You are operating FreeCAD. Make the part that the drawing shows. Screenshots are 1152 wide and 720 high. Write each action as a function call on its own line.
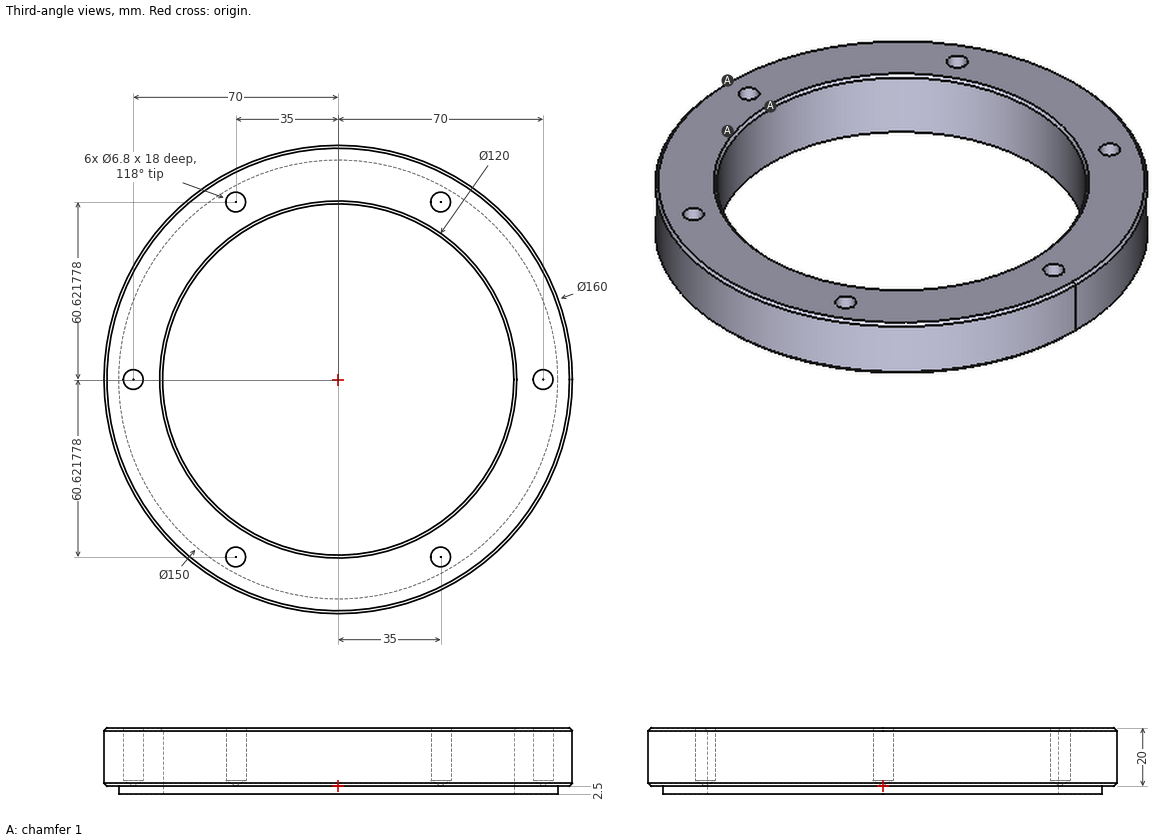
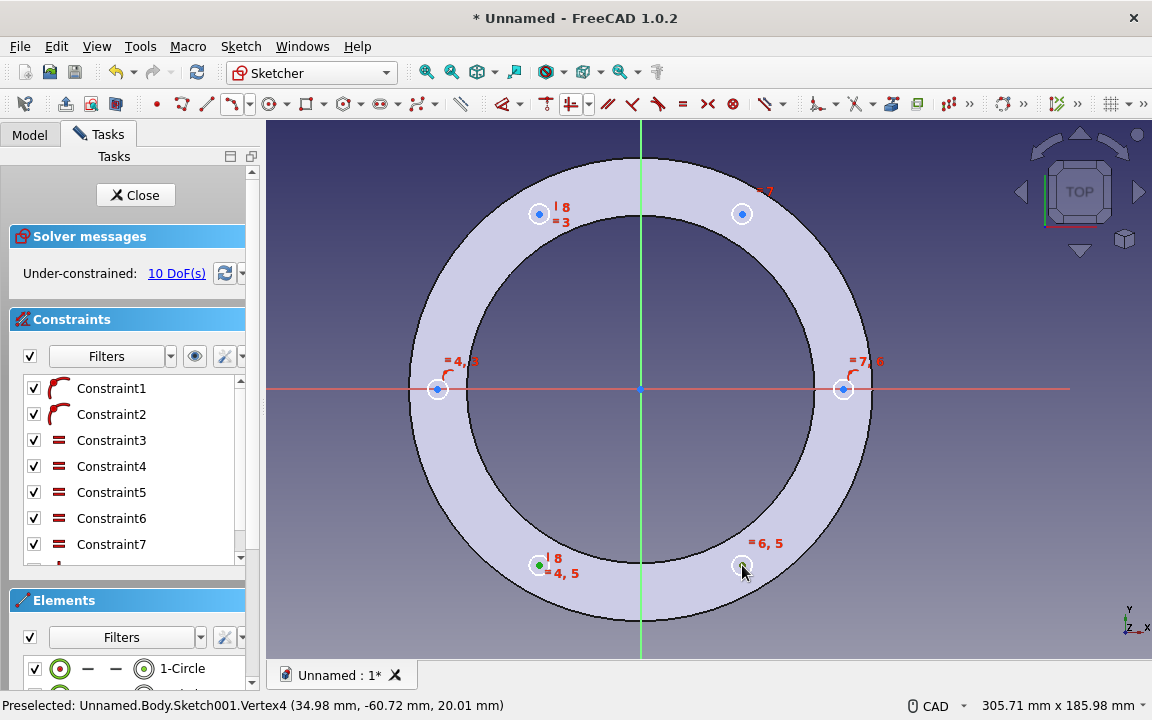
key(h)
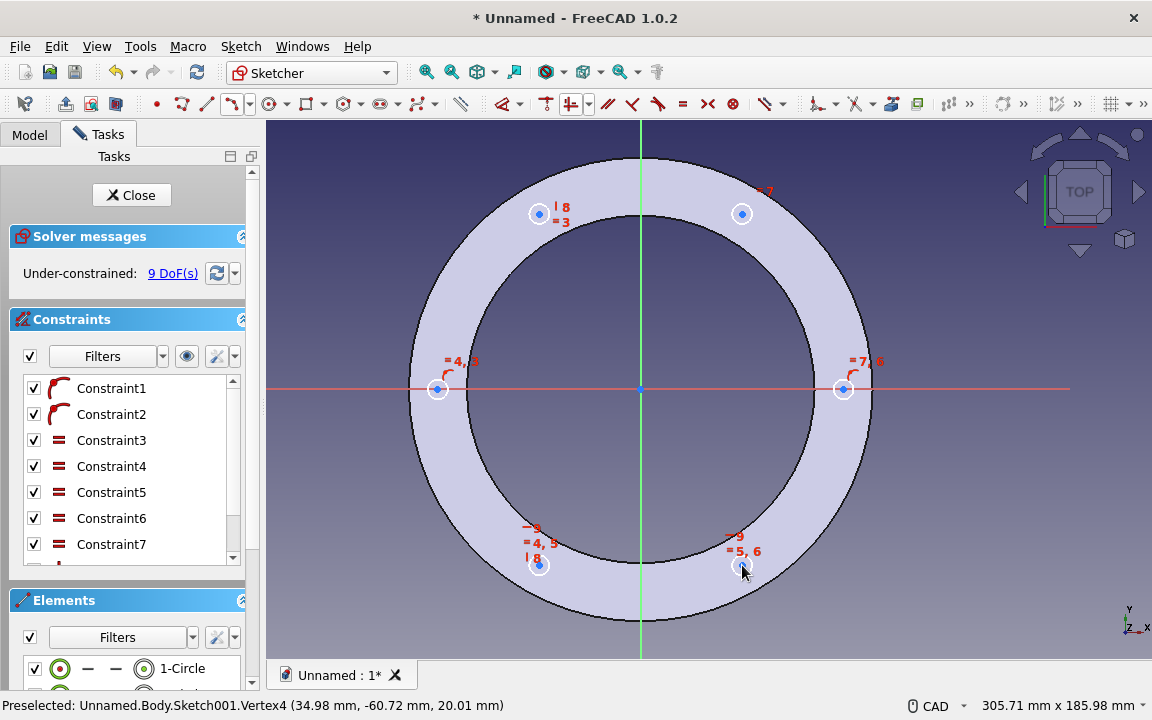
click(742, 565)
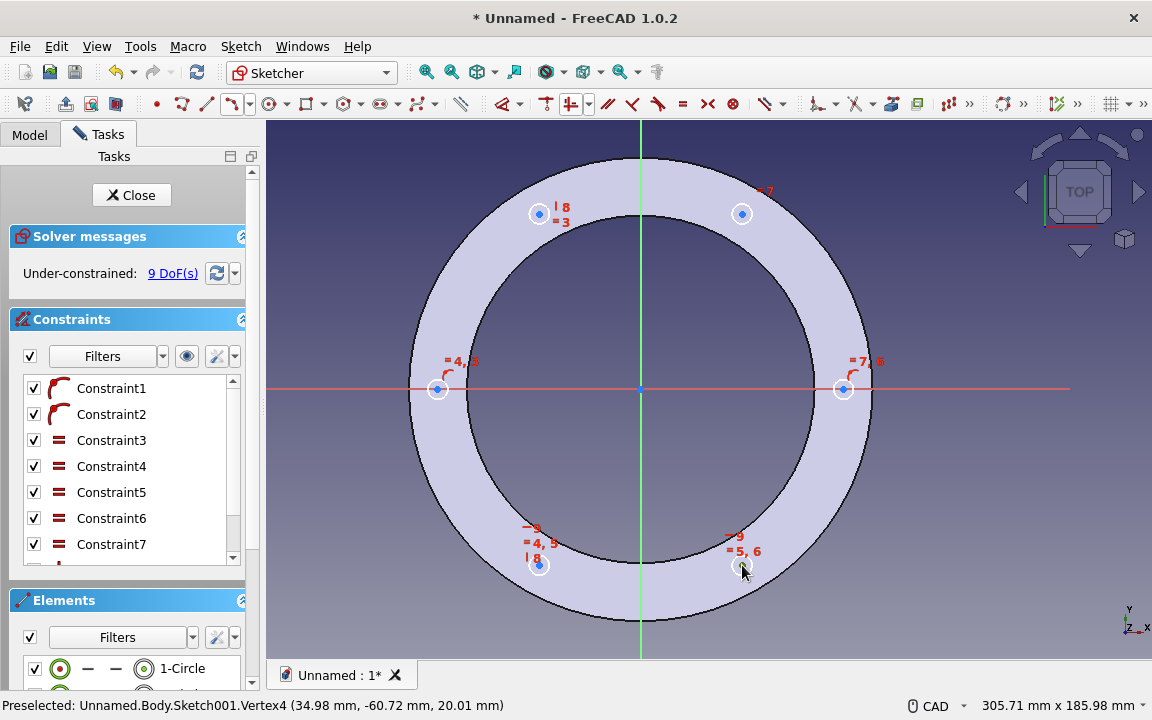
click(742, 214)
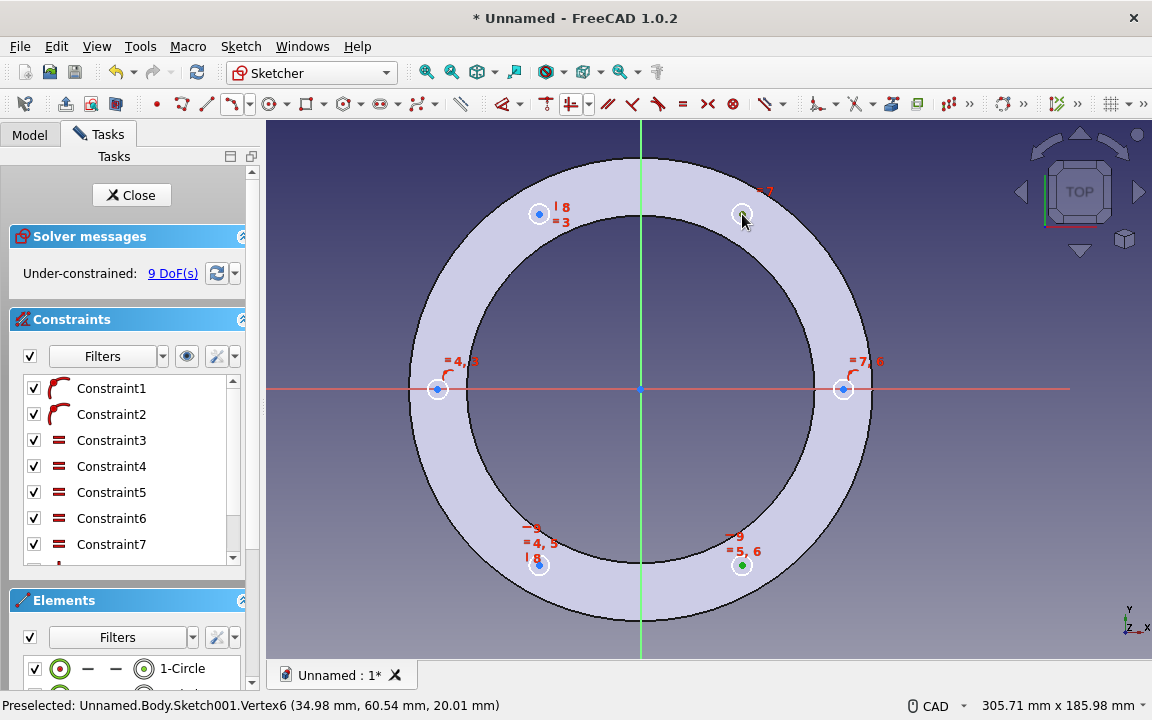
key(v)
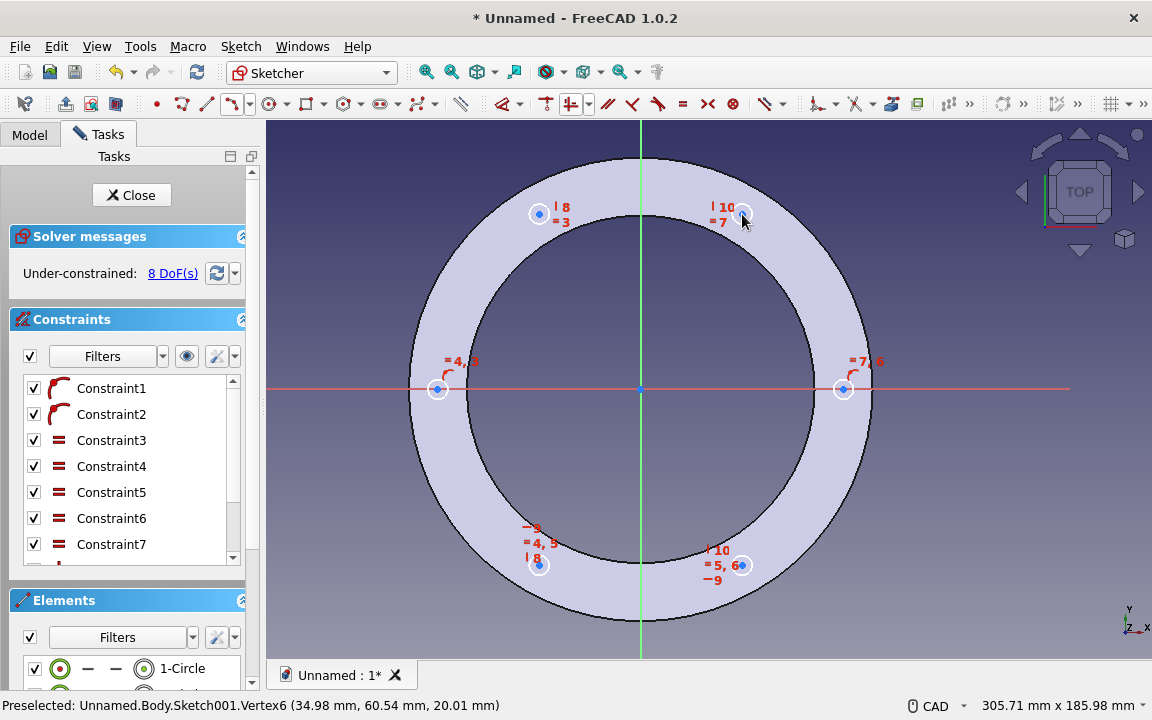
click(539, 214)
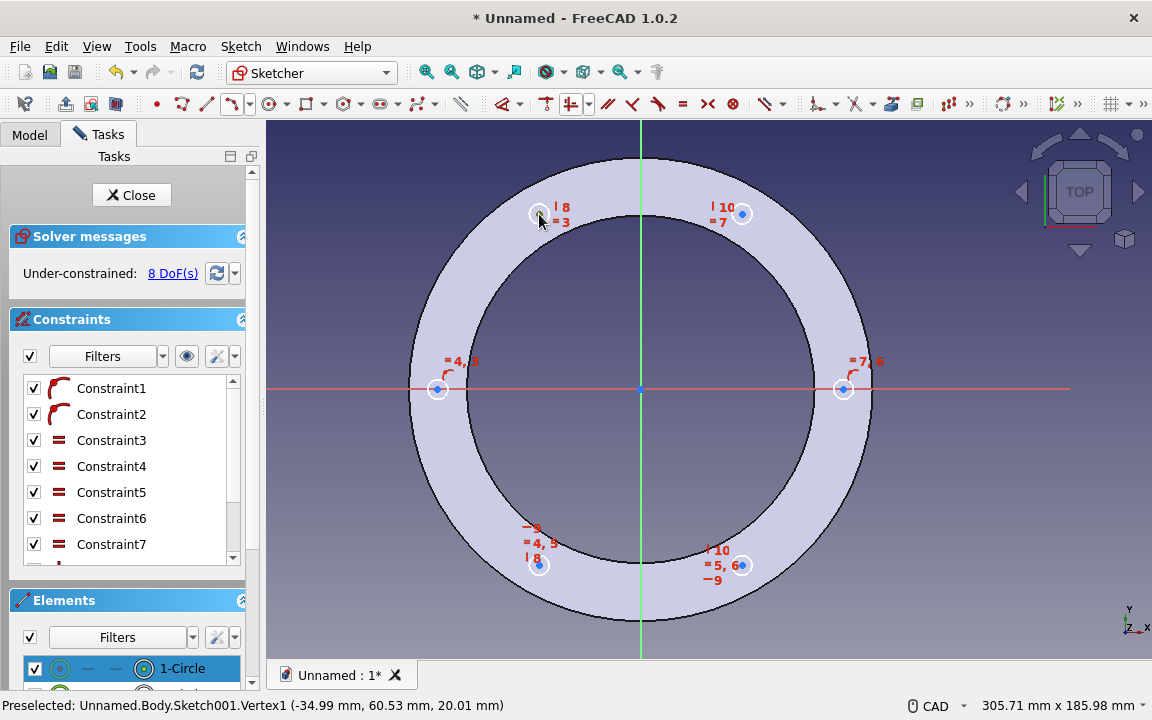
click(742, 214)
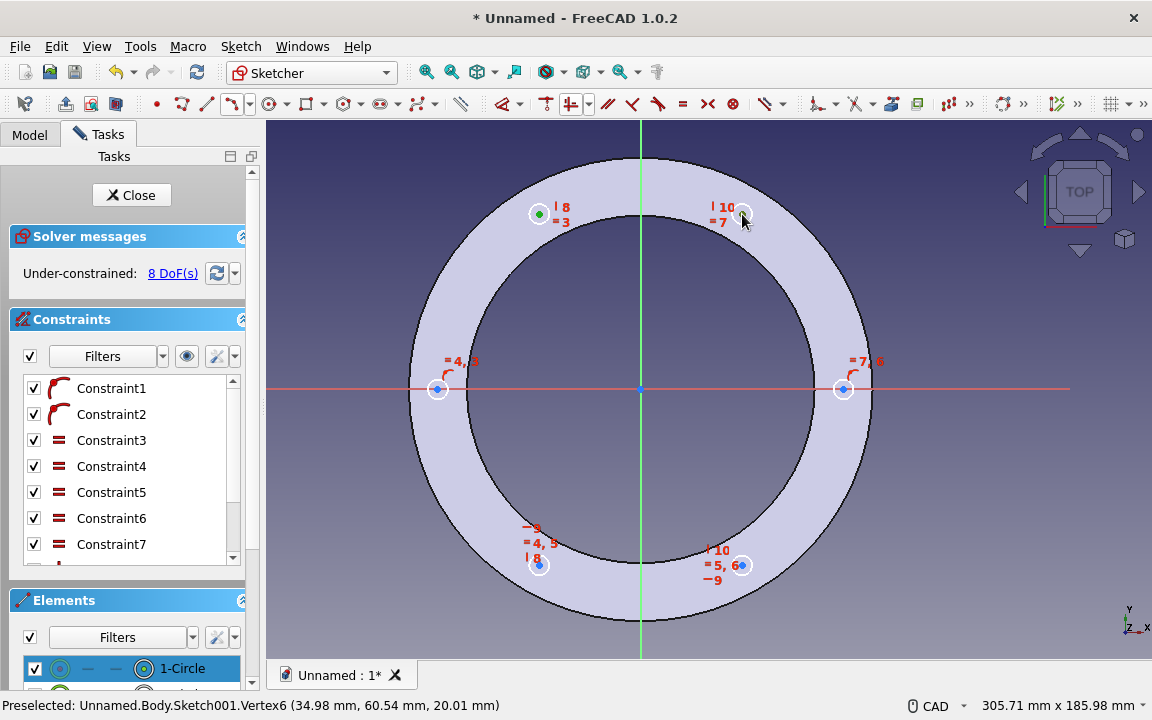
key(h)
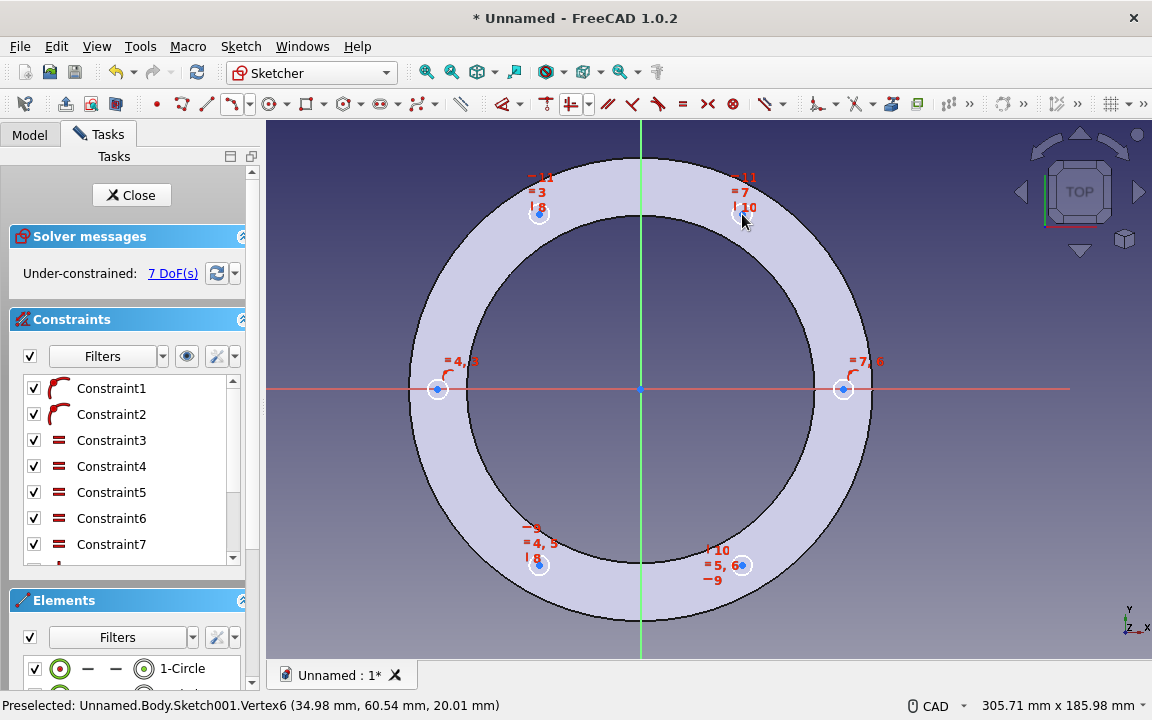
click(502, 104)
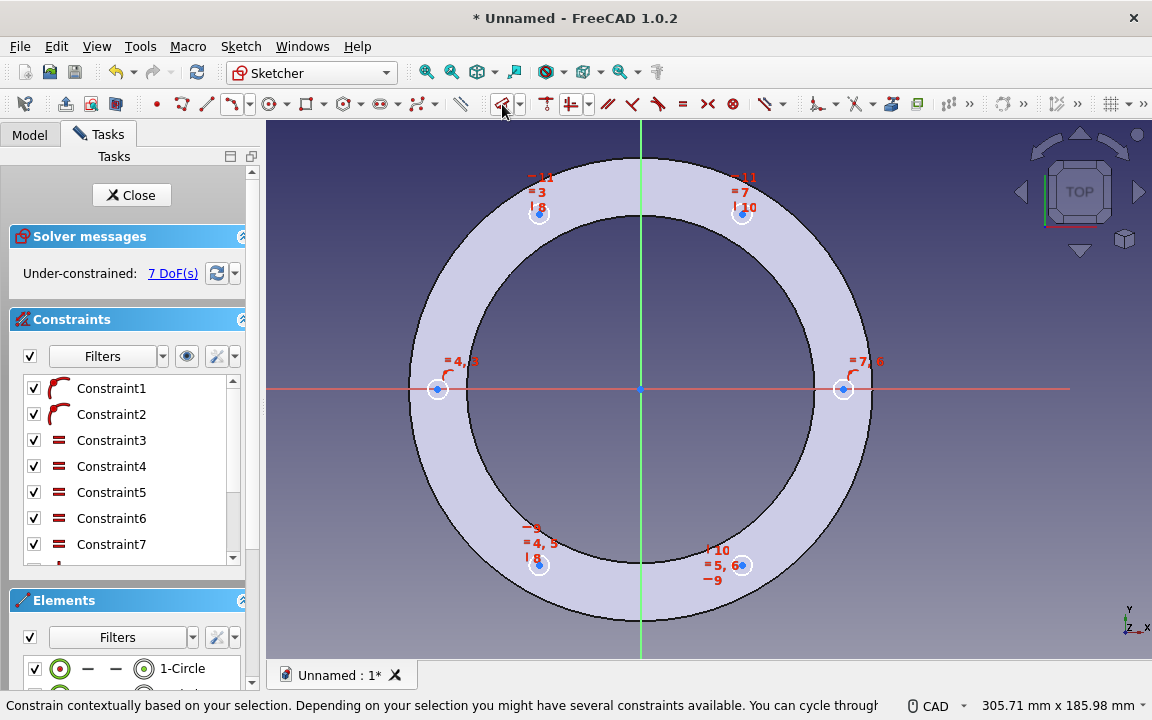
scroll(546, 207, up, 4)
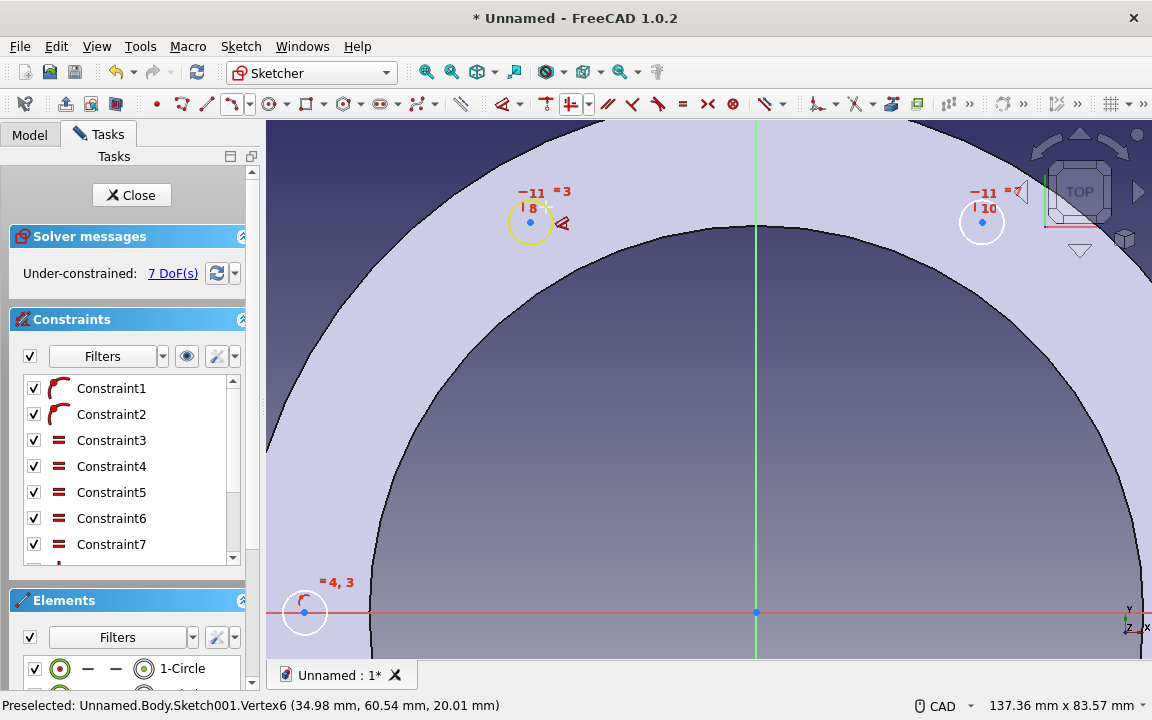
click(546, 207)
click(569, 184)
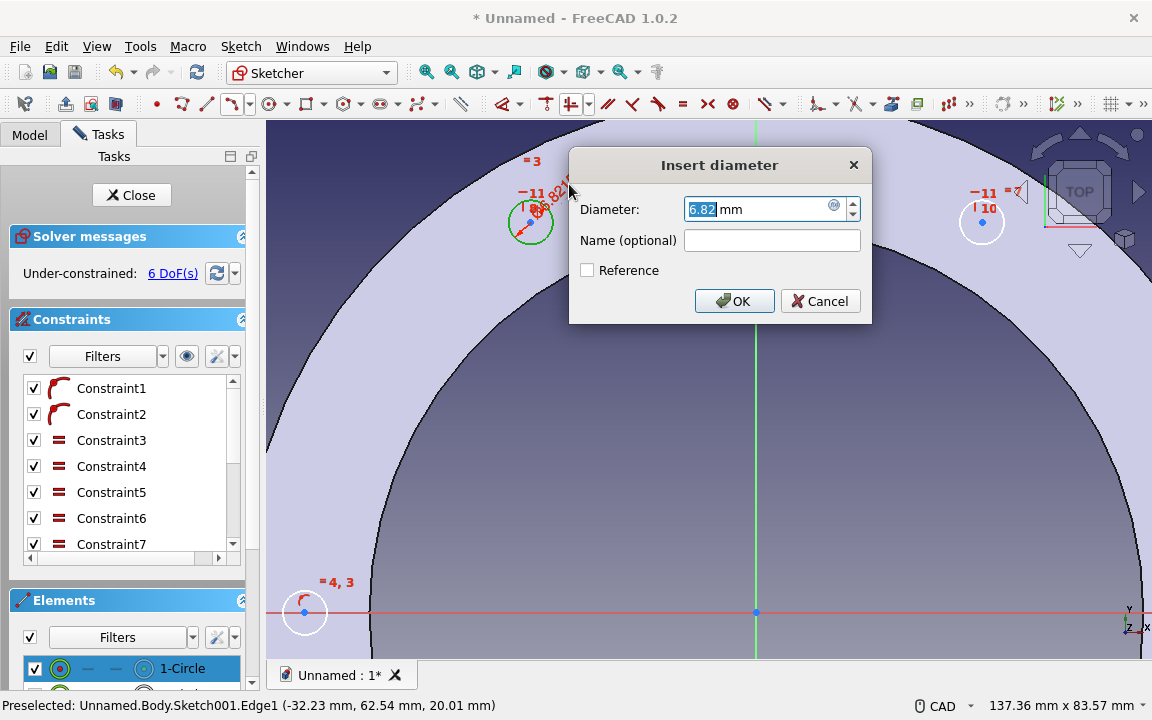
text(6.8)
key(Return)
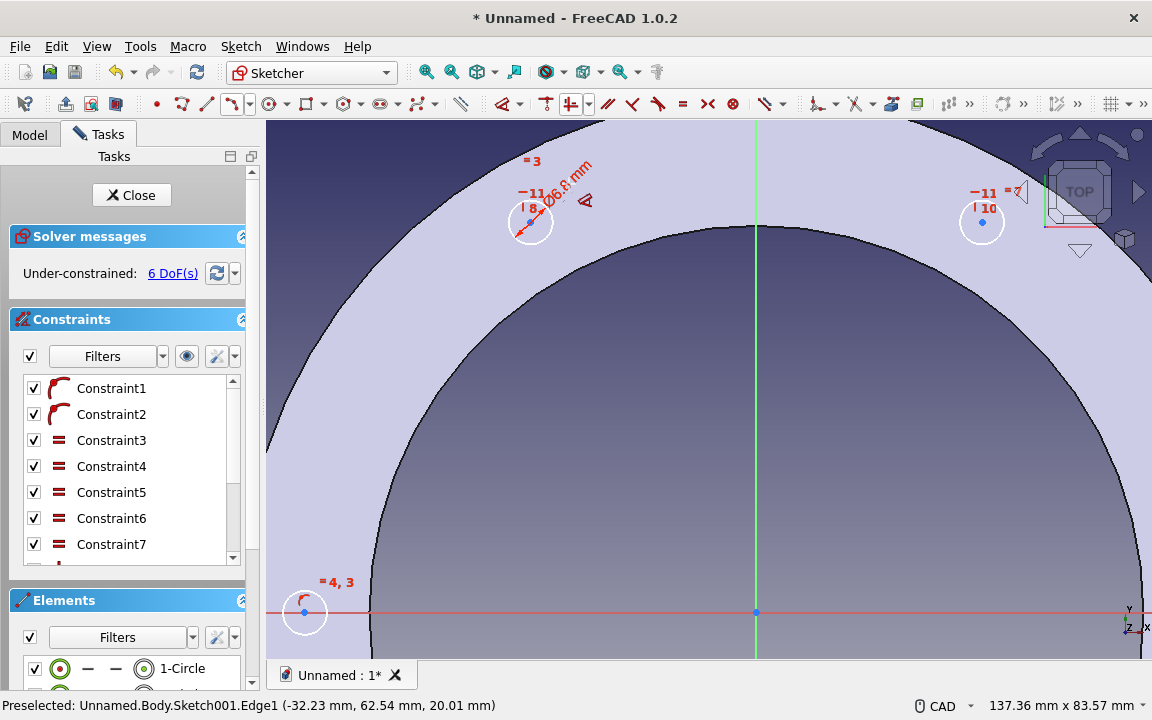
click(531, 222)
click(644, 188)